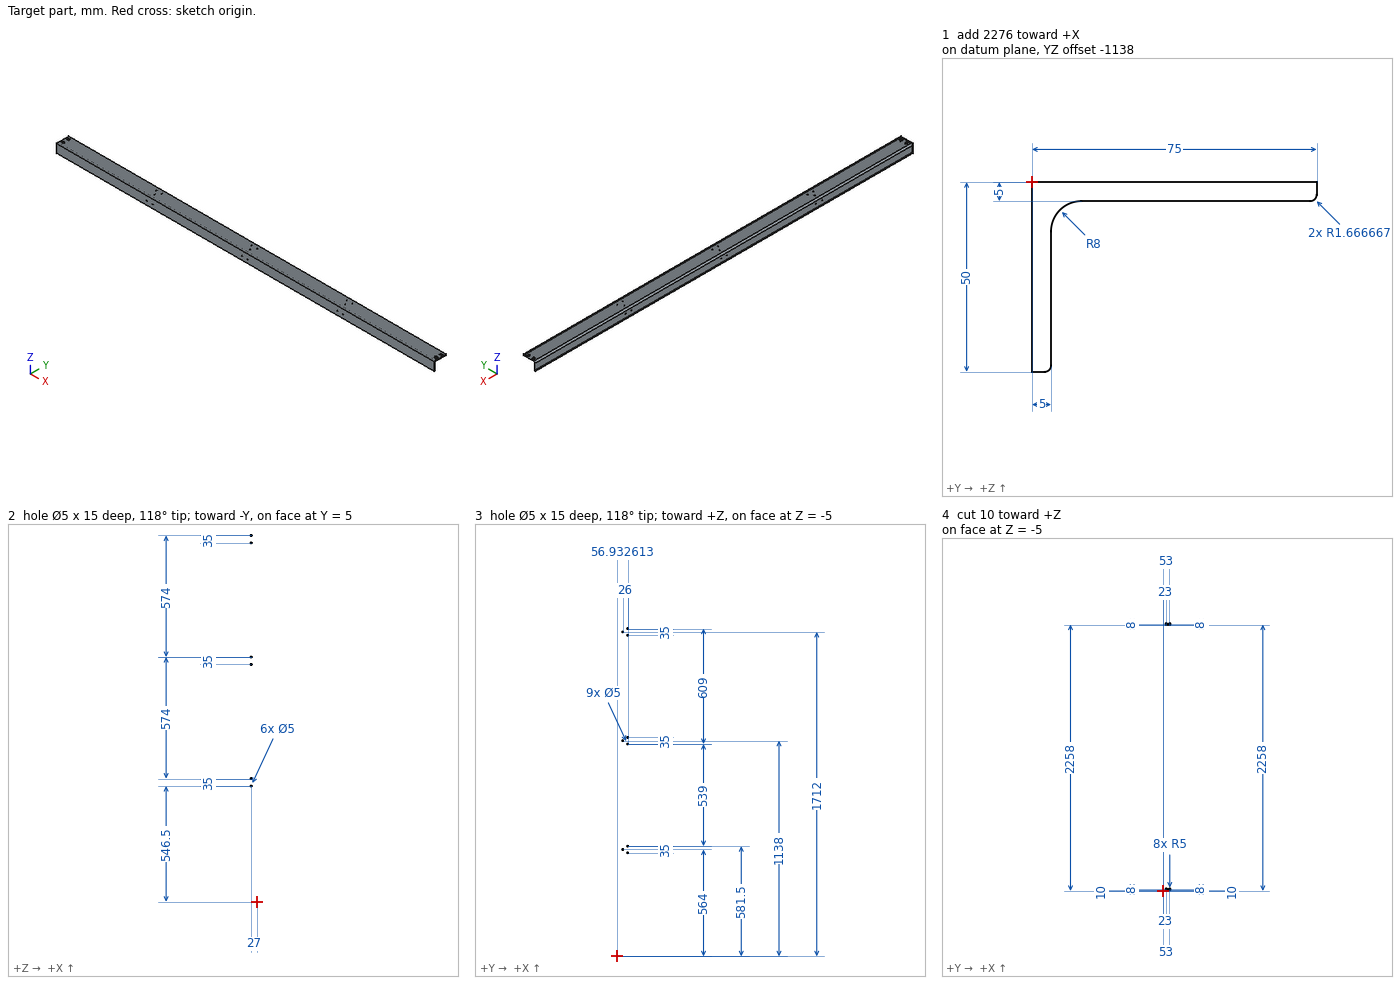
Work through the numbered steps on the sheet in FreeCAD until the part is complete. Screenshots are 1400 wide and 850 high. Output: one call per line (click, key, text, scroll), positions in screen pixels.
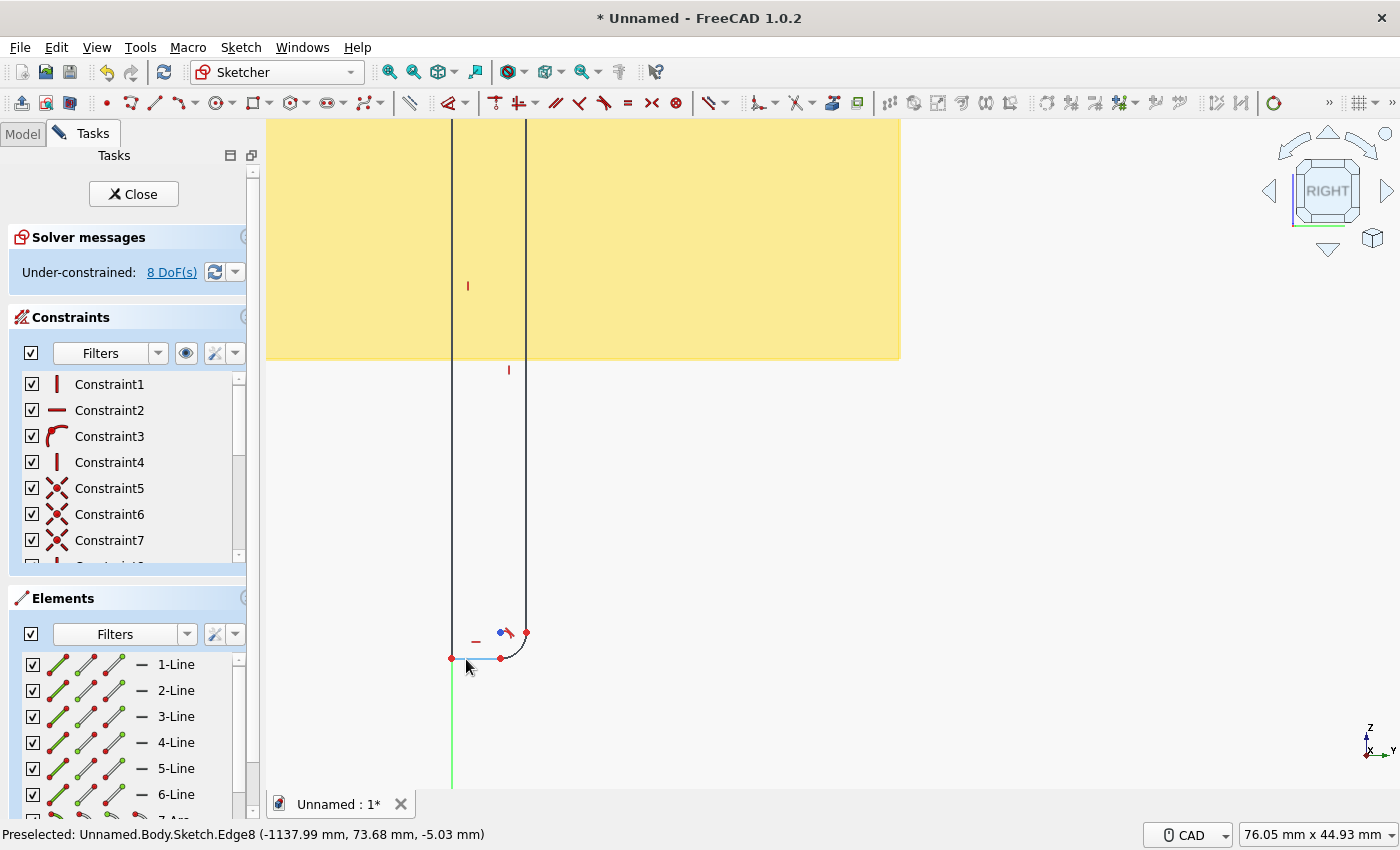
click(466, 659)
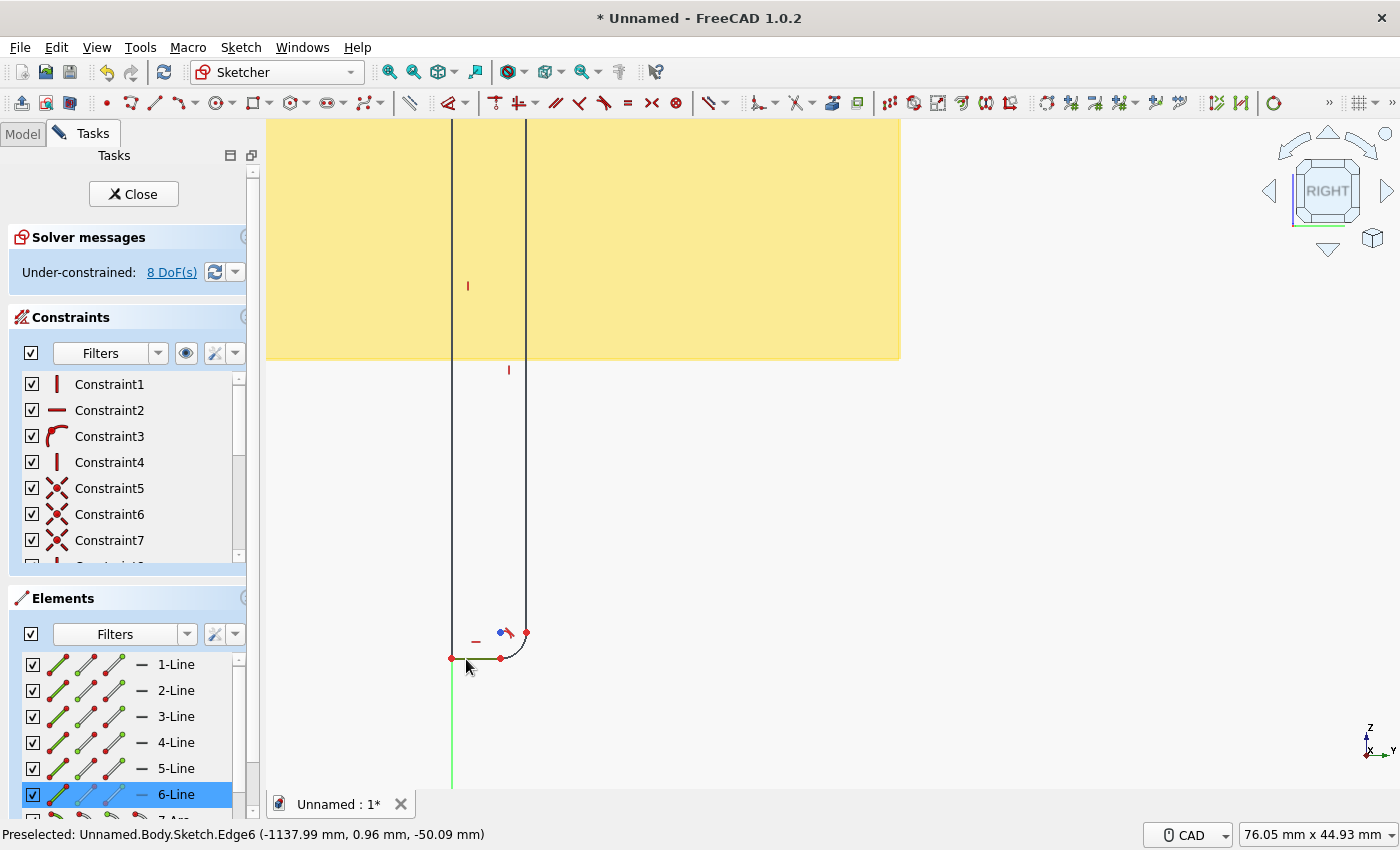
click(512, 656)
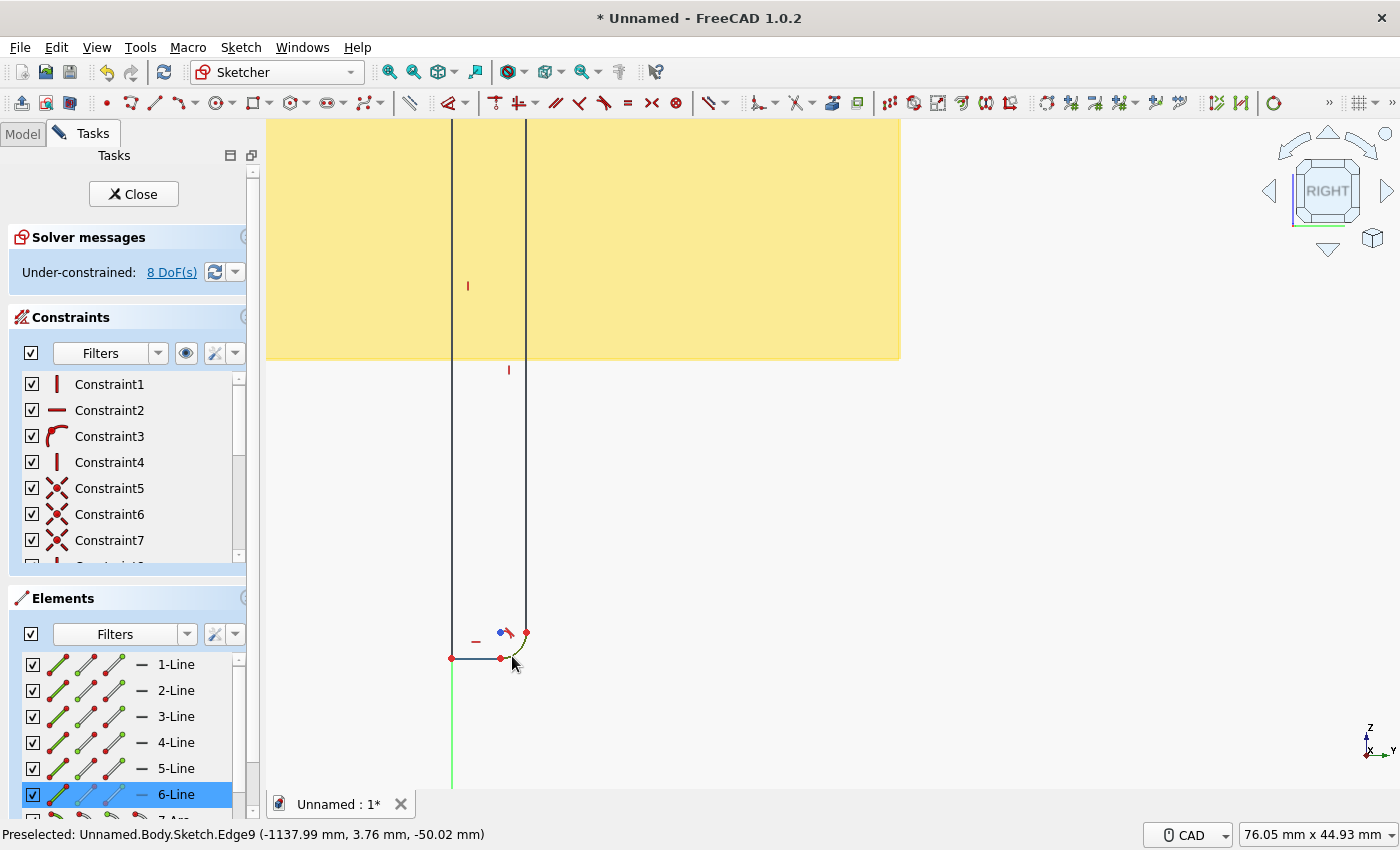
click(604, 104)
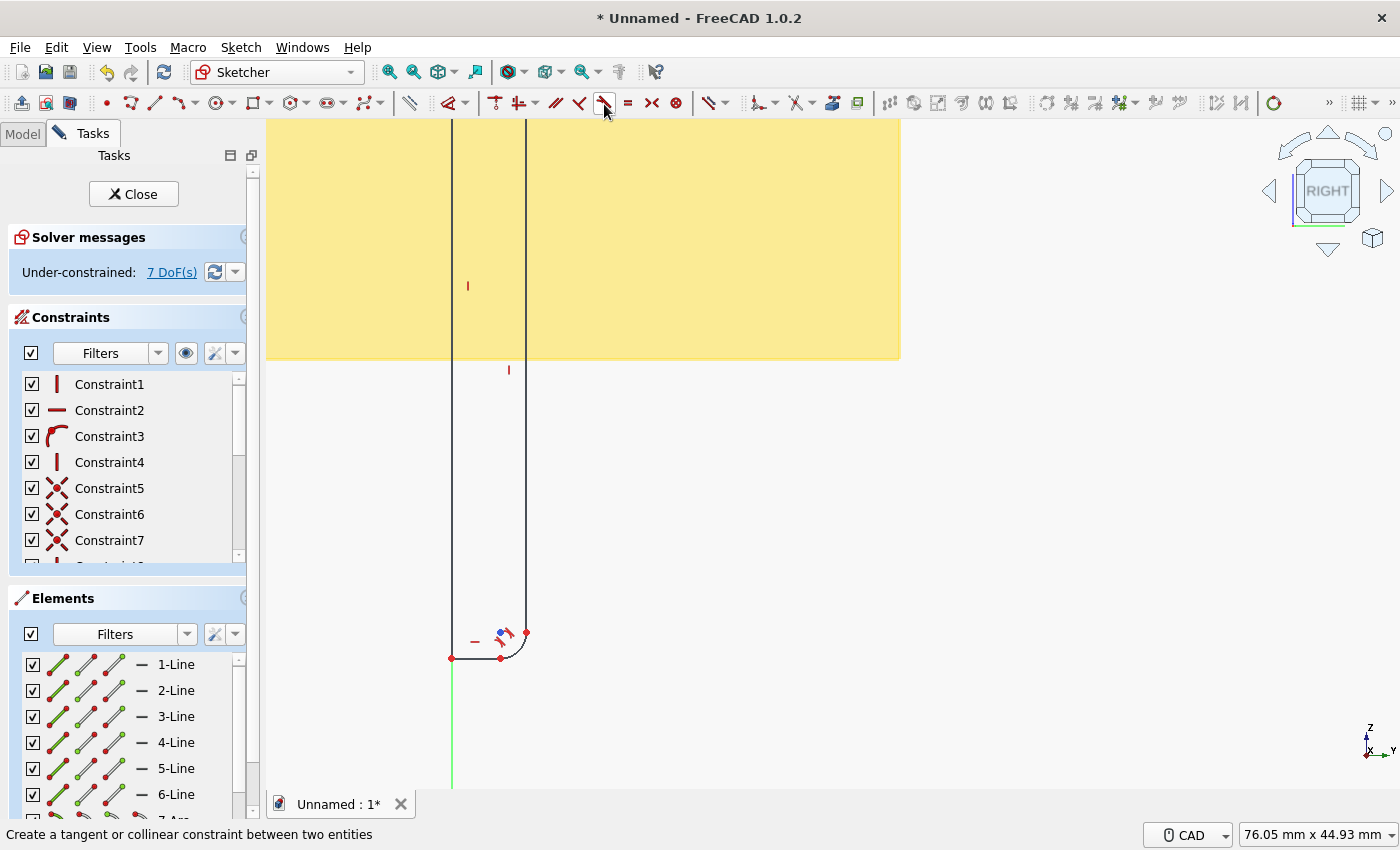
scroll(465, 660, down, 3)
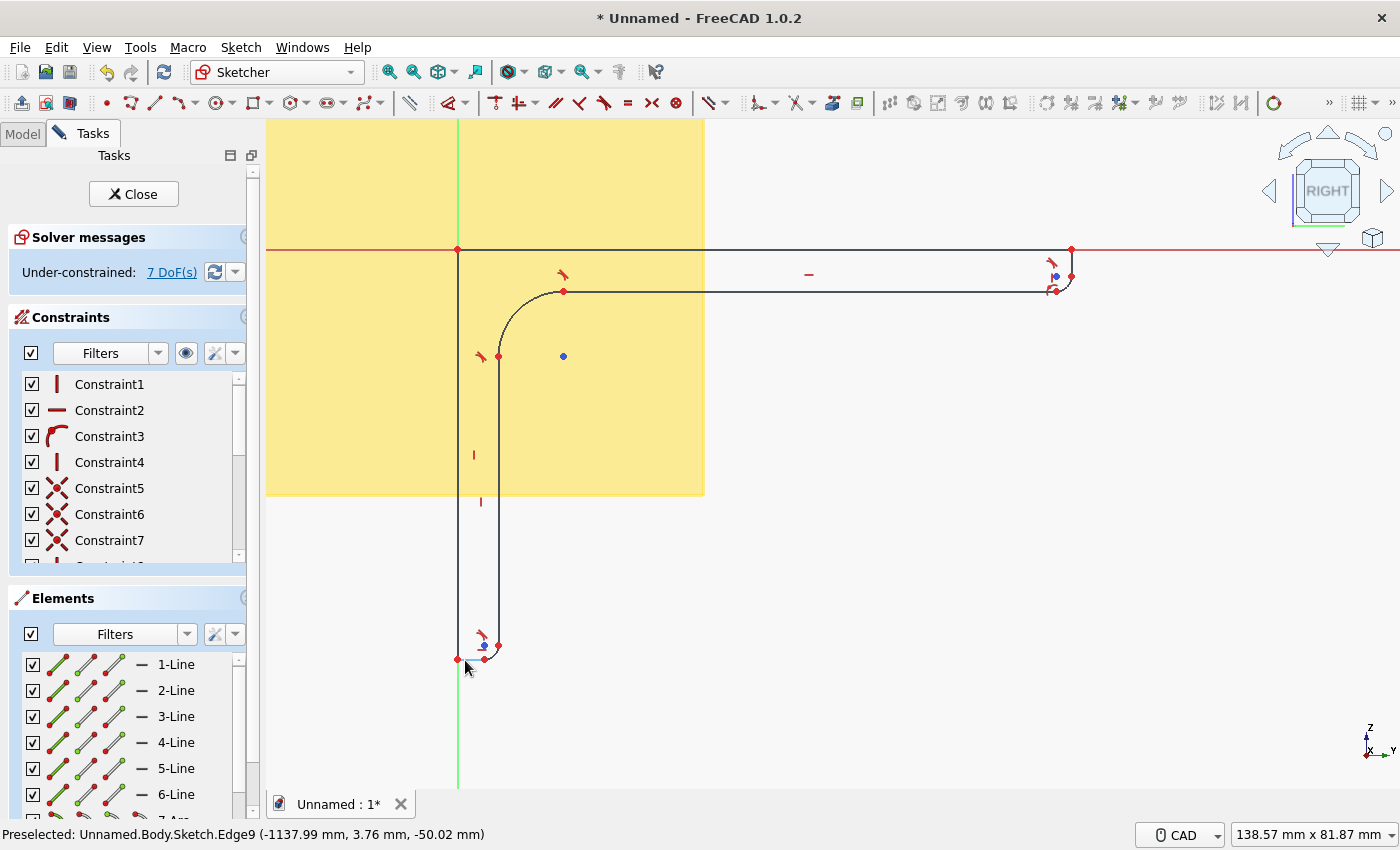
scroll(1063, 290, up, 4)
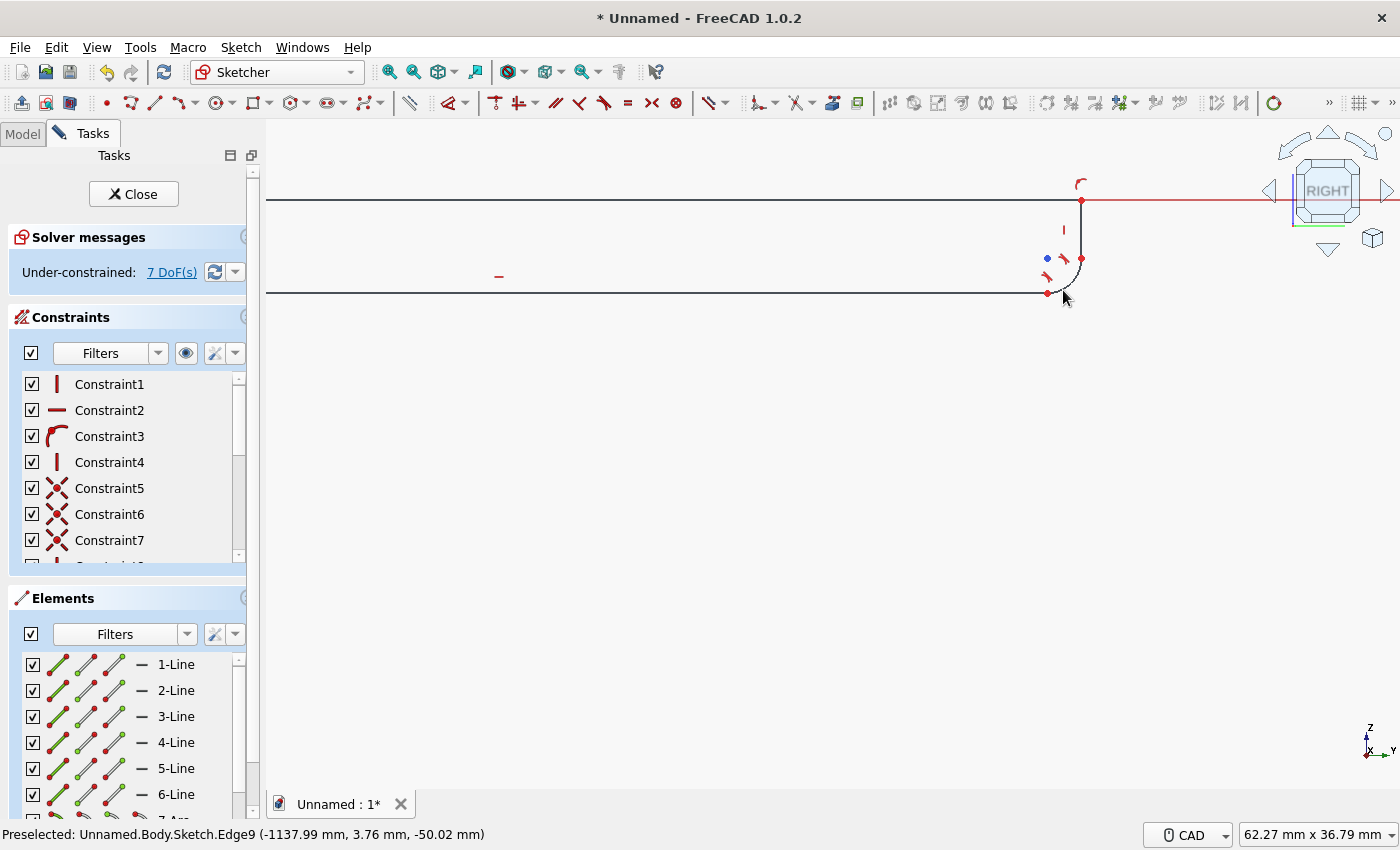
click(1063, 289)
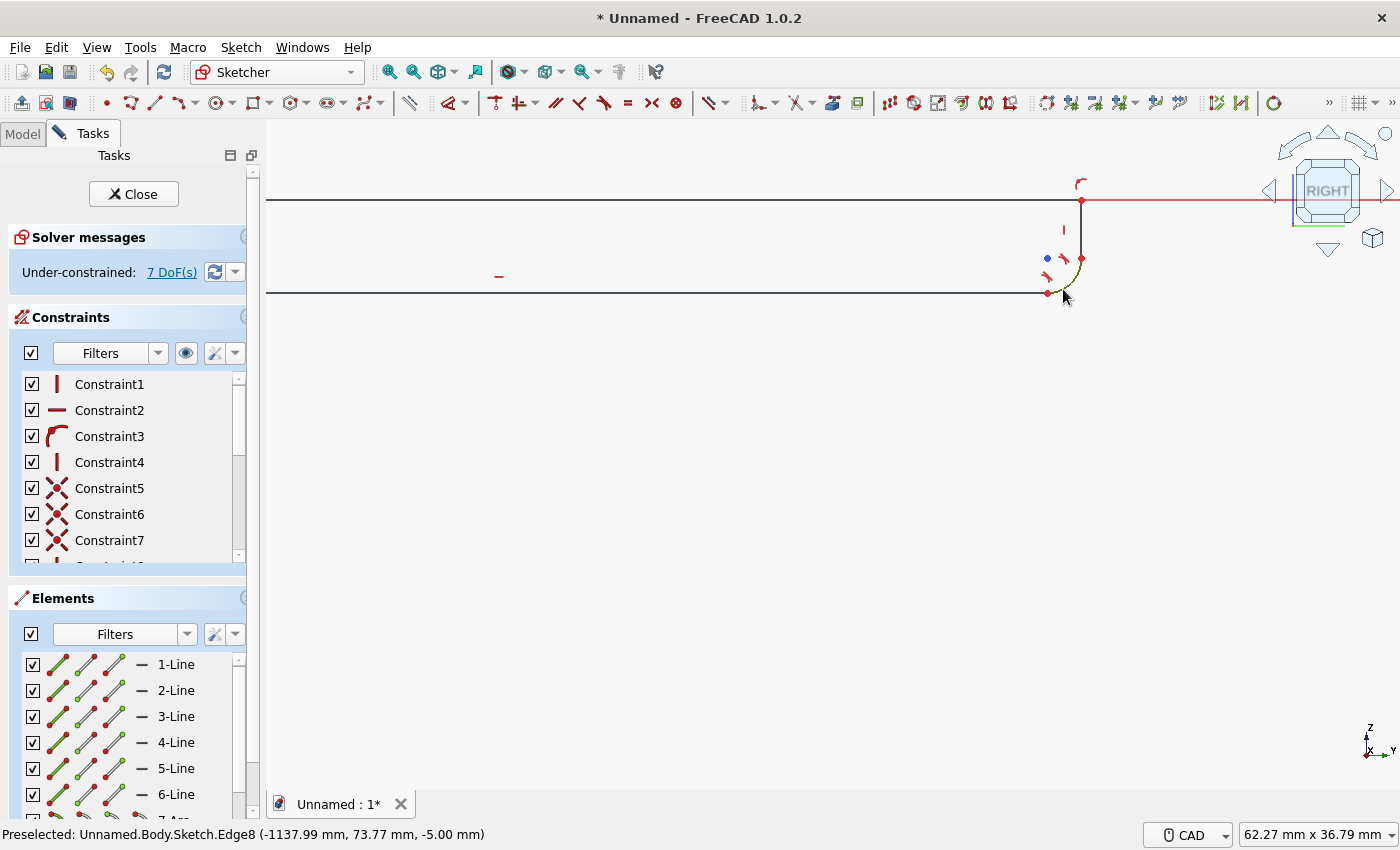
scroll(1063, 290, down, 4)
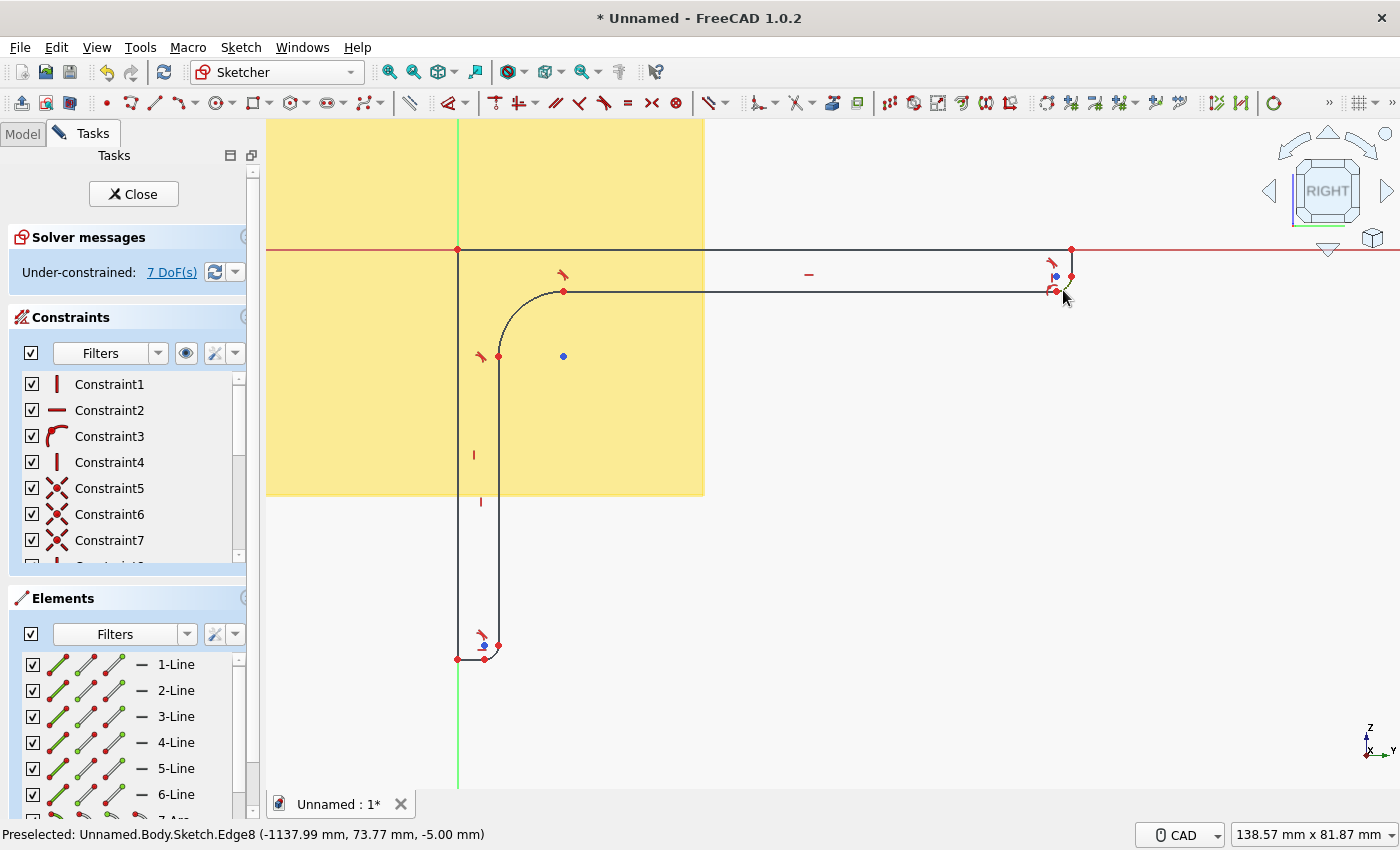
scroll(491, 658, up, 4)